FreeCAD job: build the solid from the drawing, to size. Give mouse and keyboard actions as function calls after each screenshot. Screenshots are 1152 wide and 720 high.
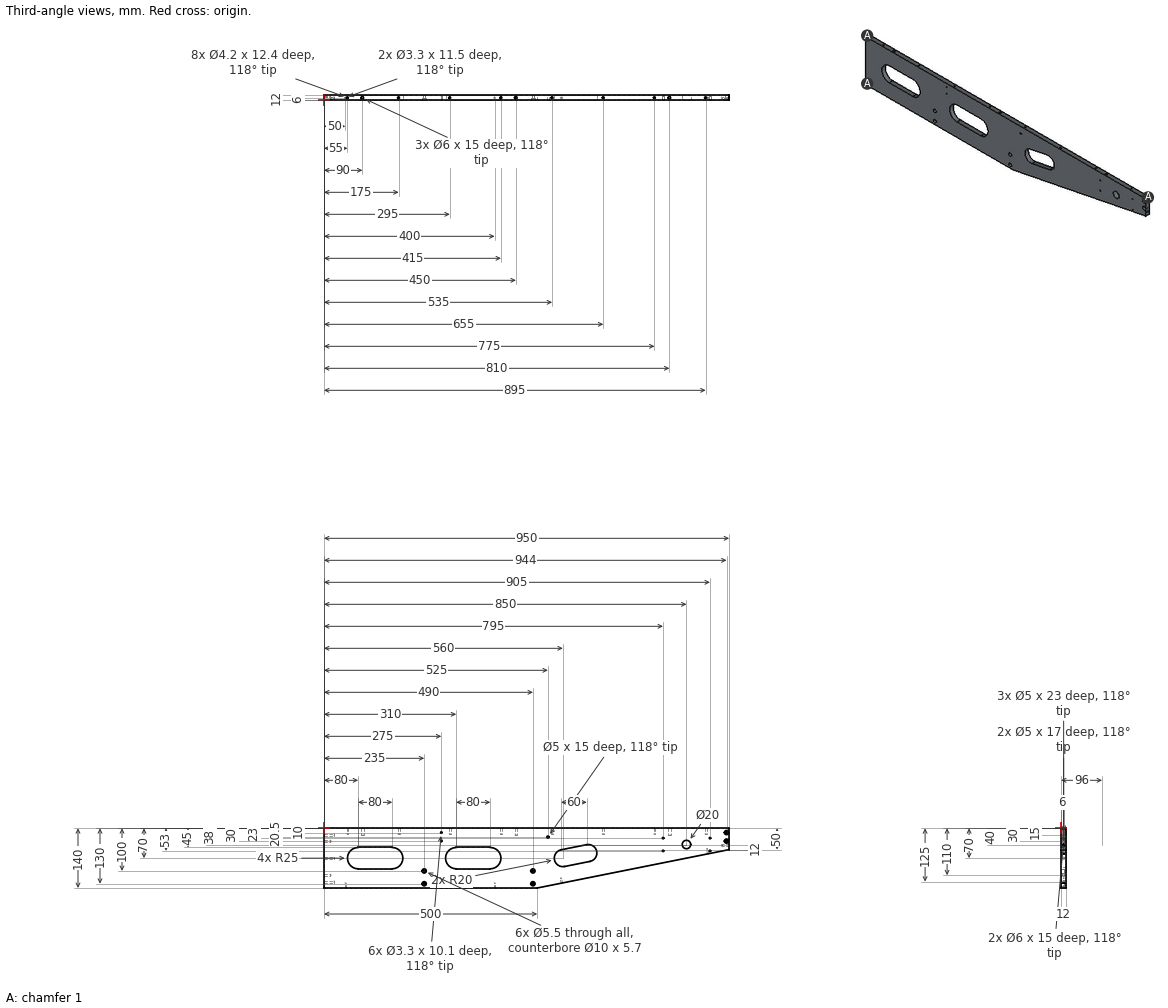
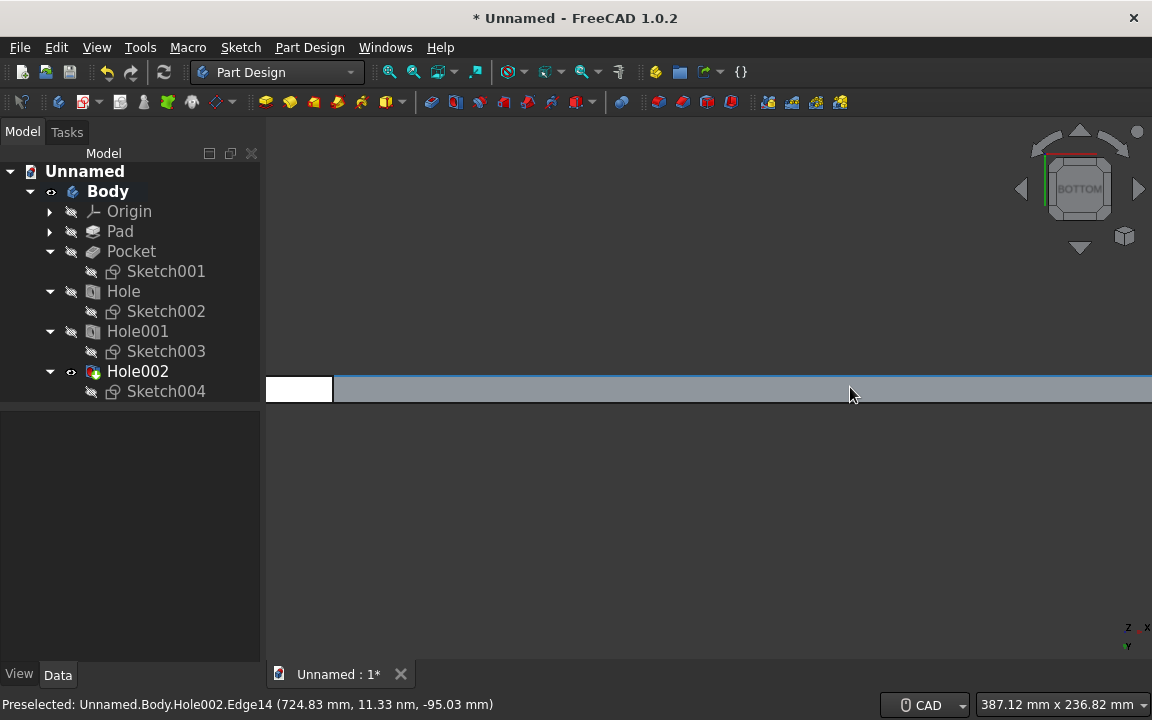
click(848, 389)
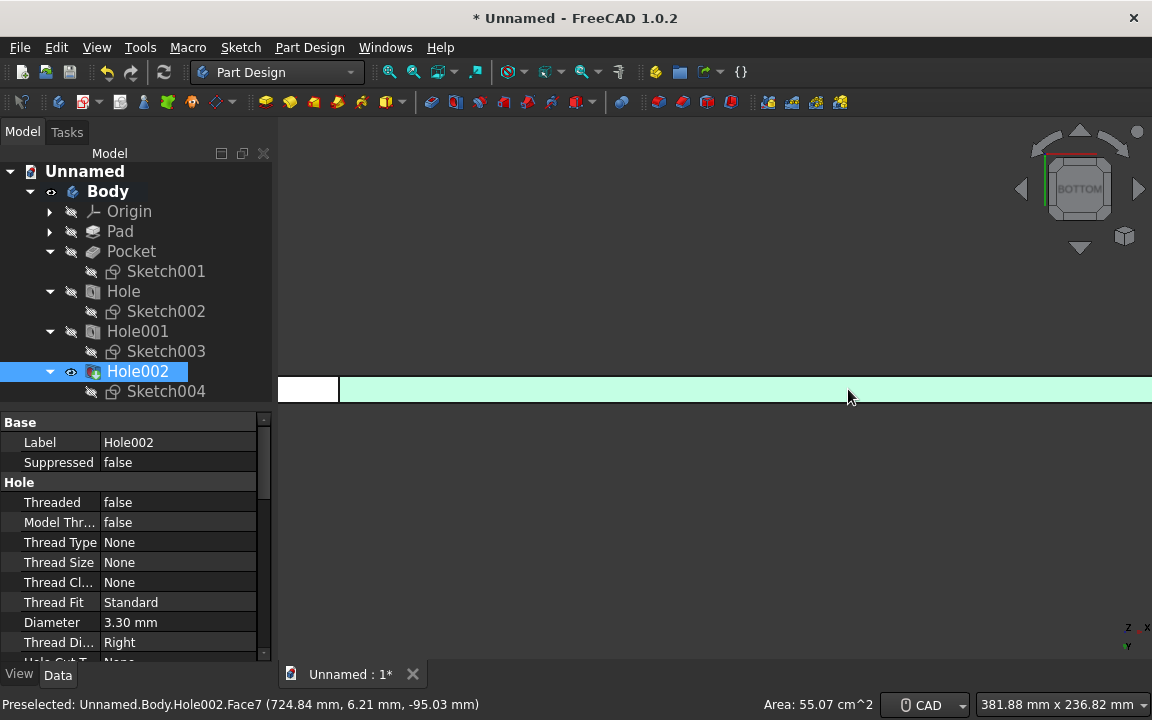
click(84, 102)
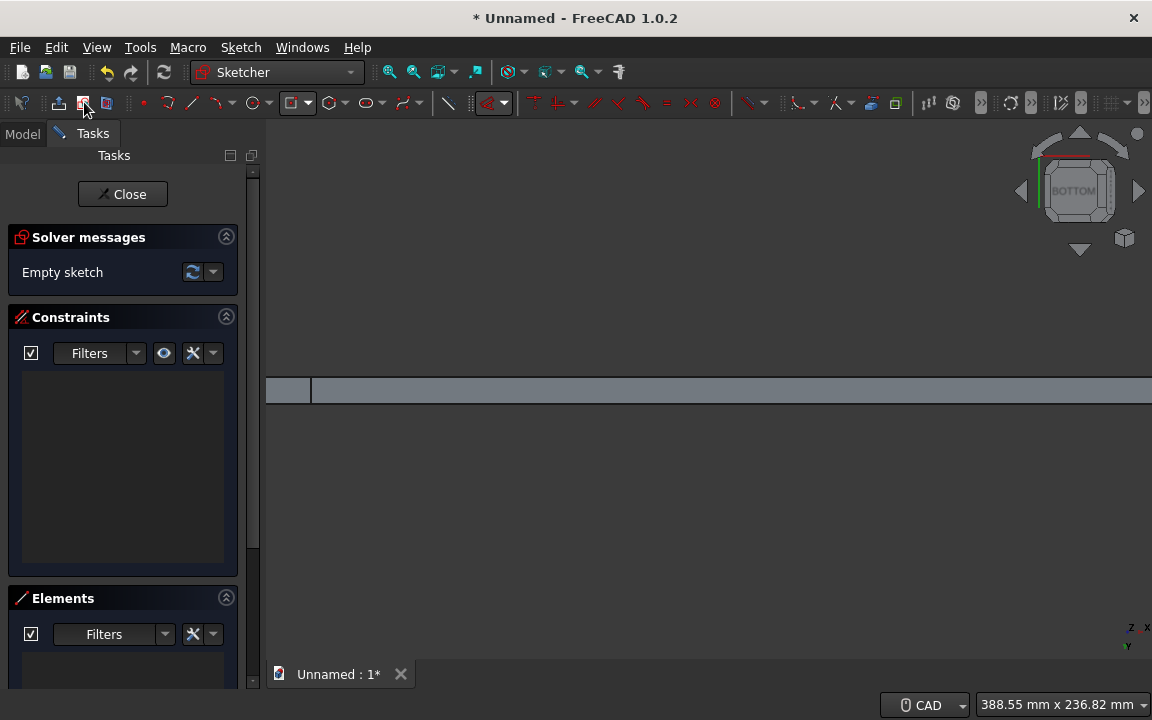
scroll(768, 390, down, 7)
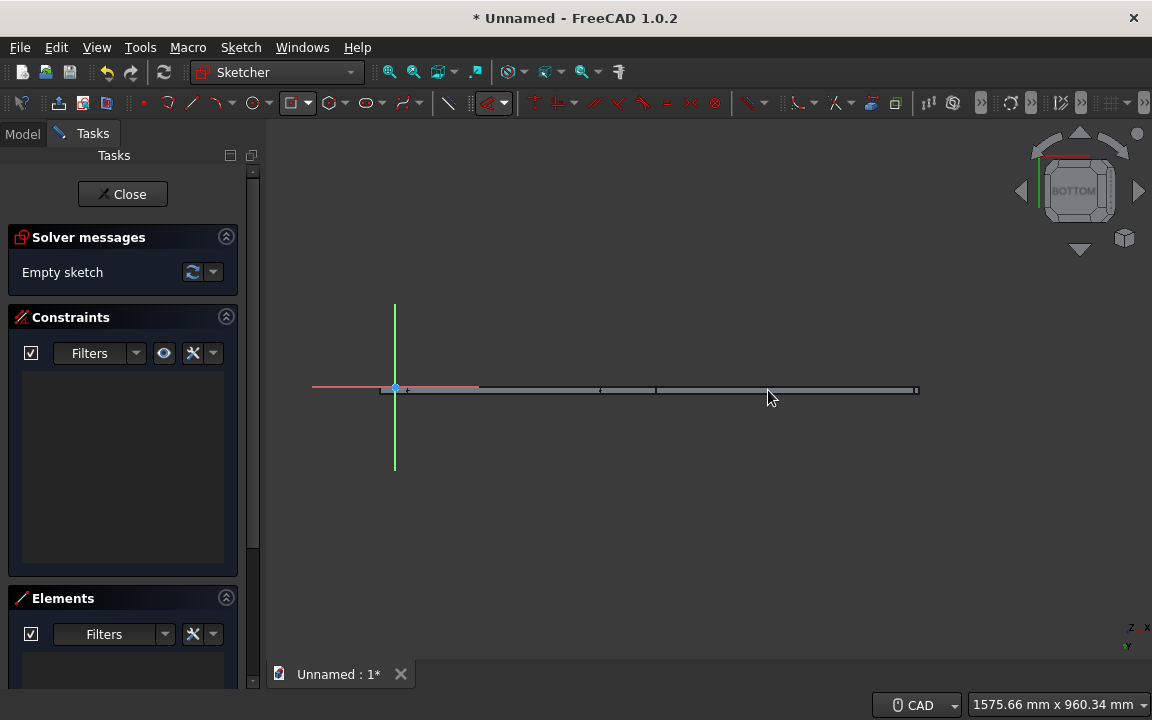
key(g)
key(c)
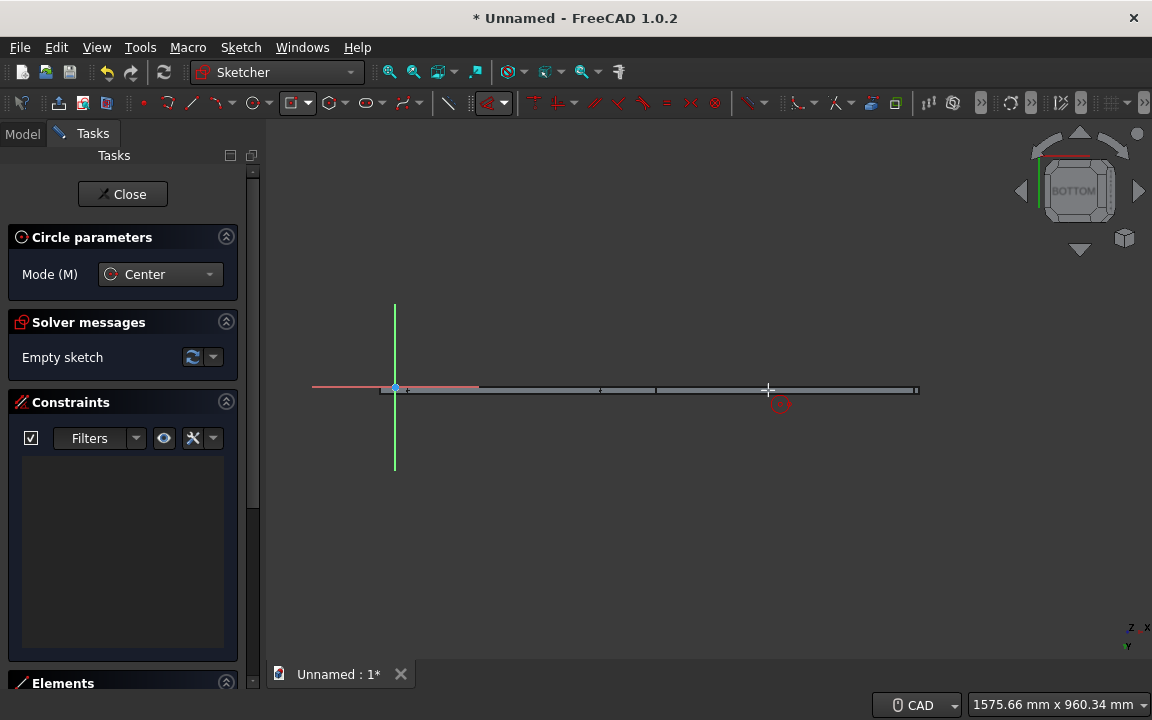
scroll(886, 391, up, 16)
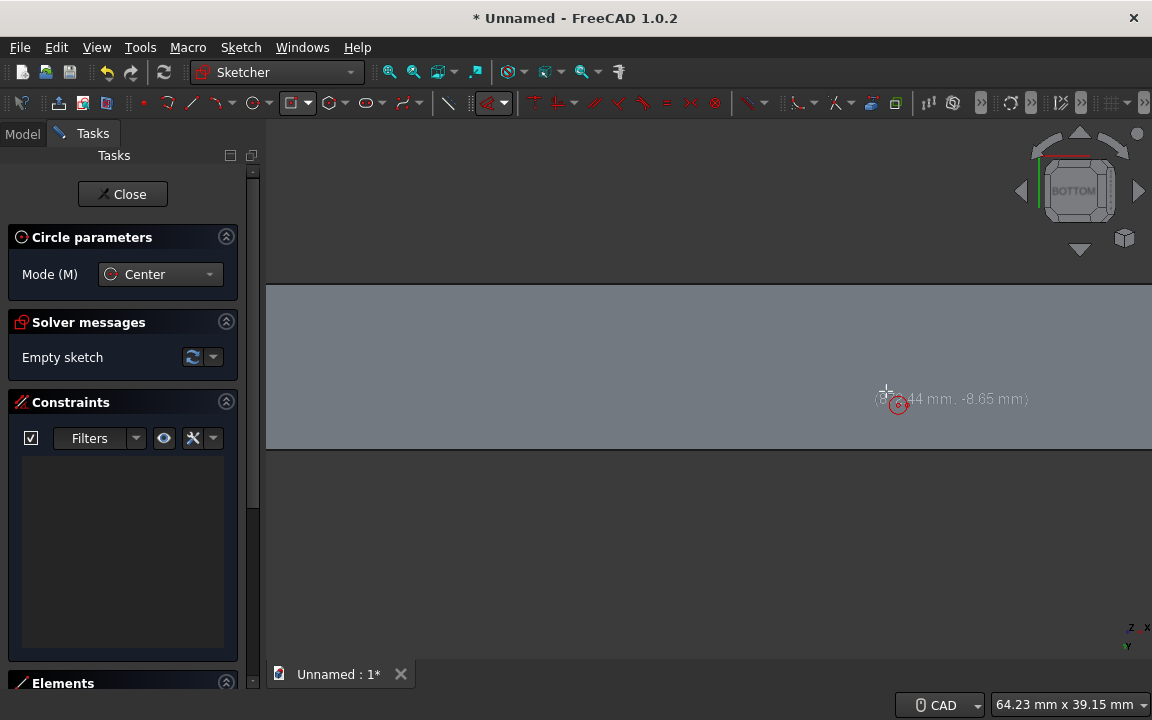
scroll(943, 392, down, 15)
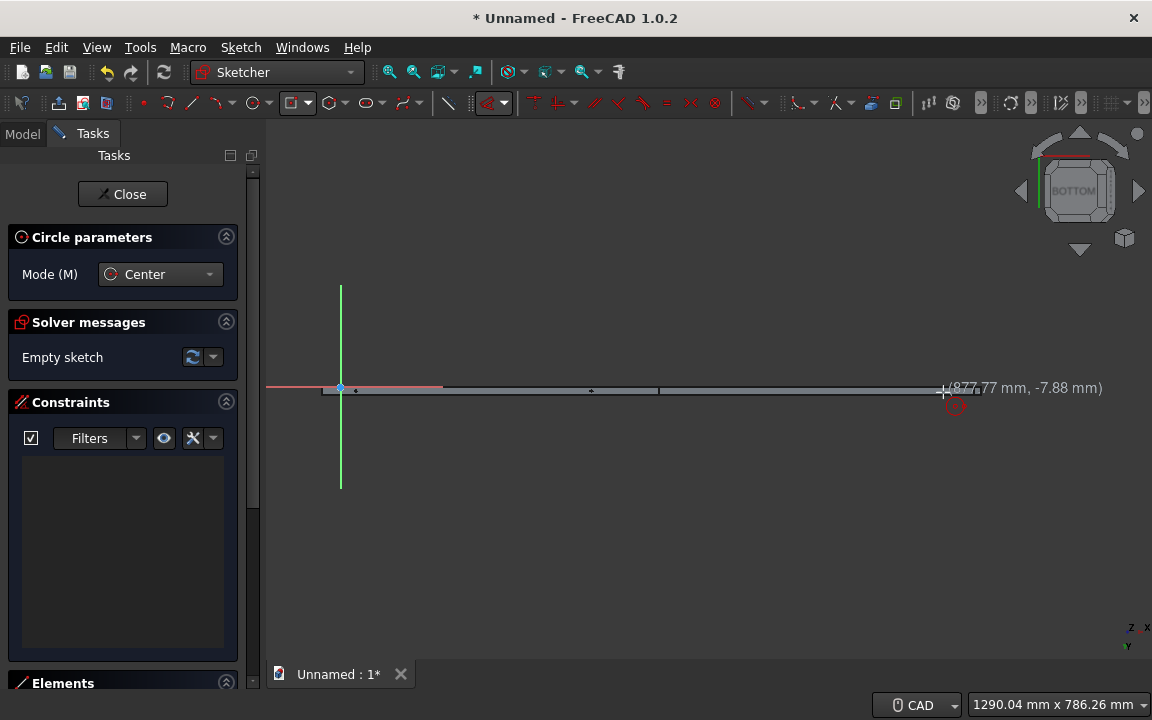
scroll(940, 391, up, 7)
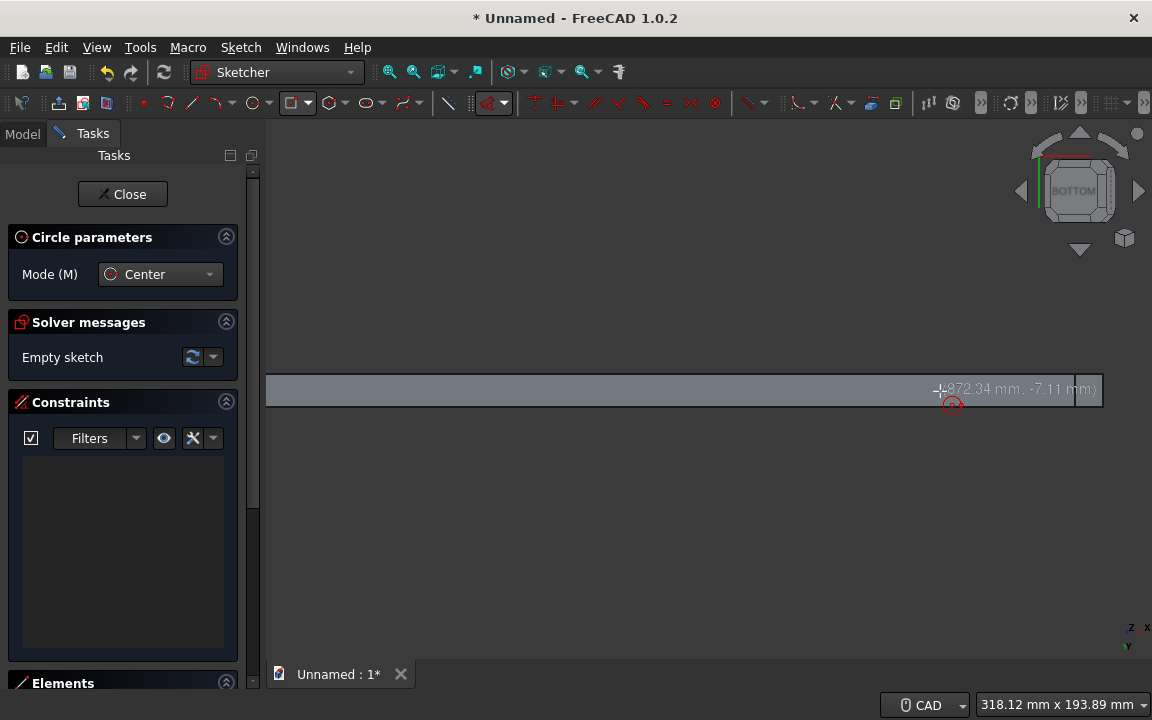
click(936, 390)
move(939, 394)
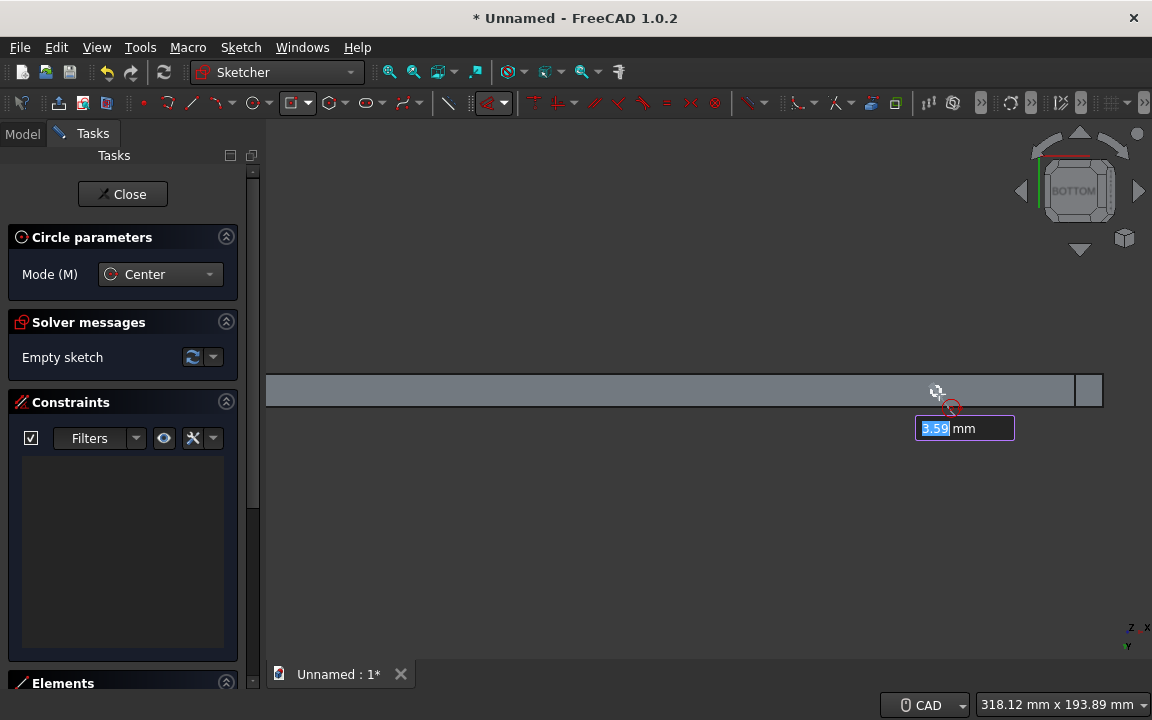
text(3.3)
key(Return)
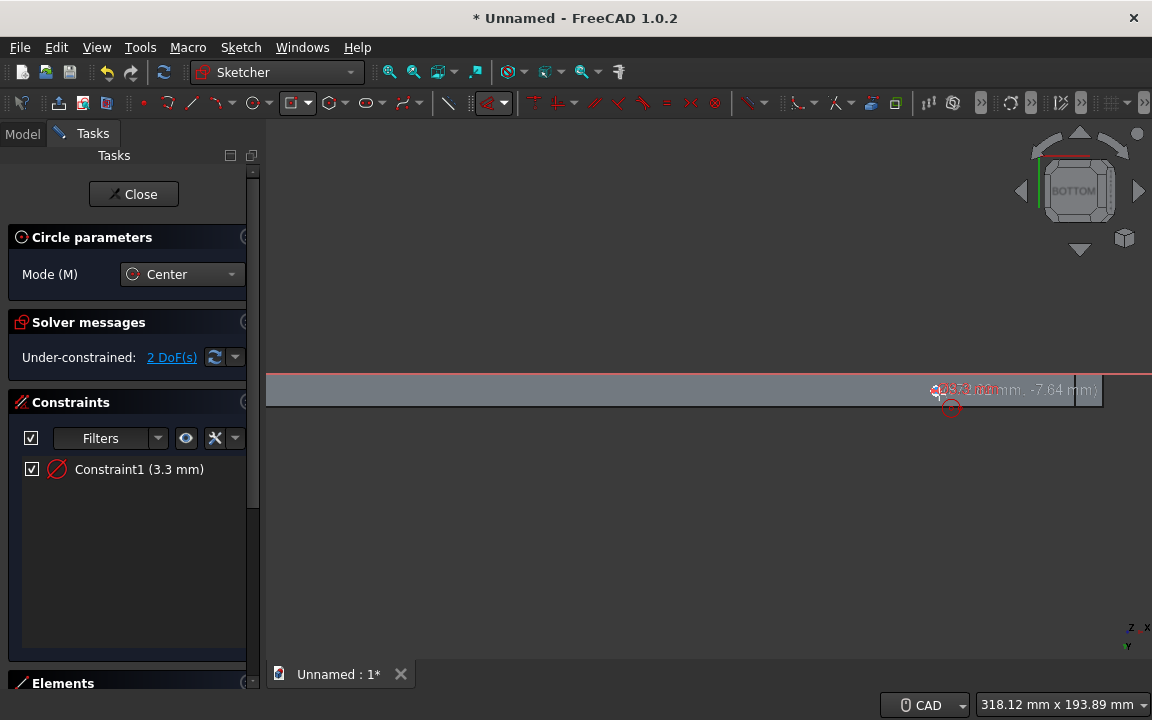
scroll(872, 390, down, 8)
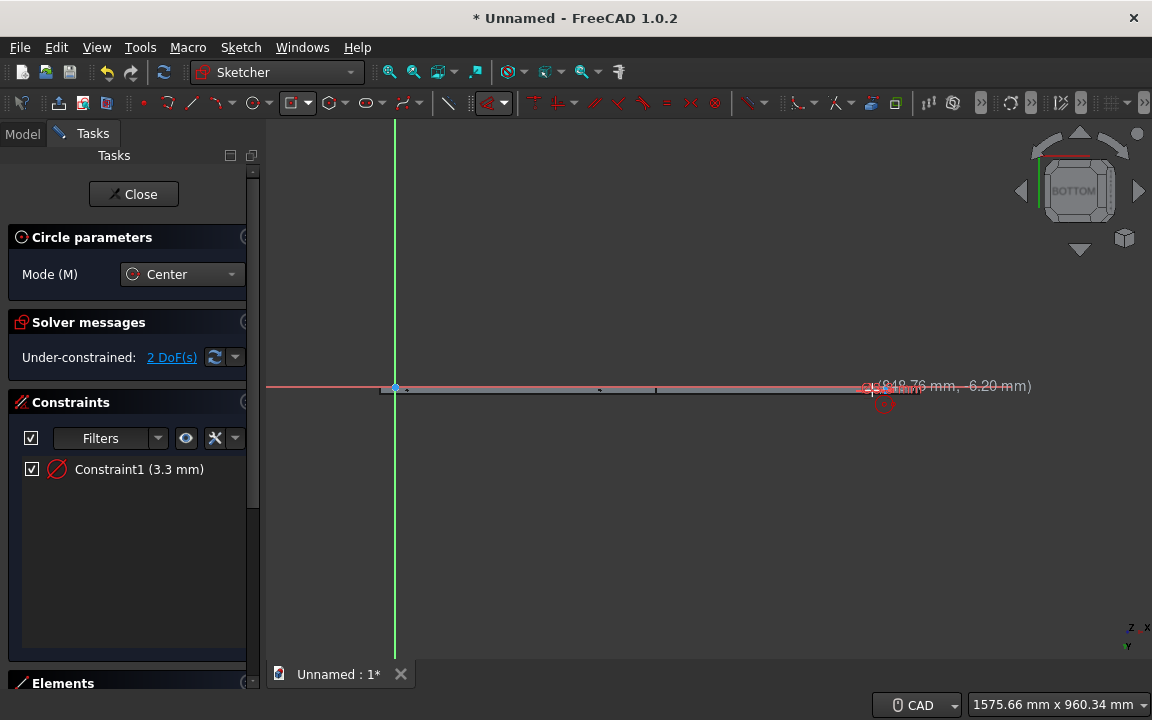
scroll(689, 390, up, 16)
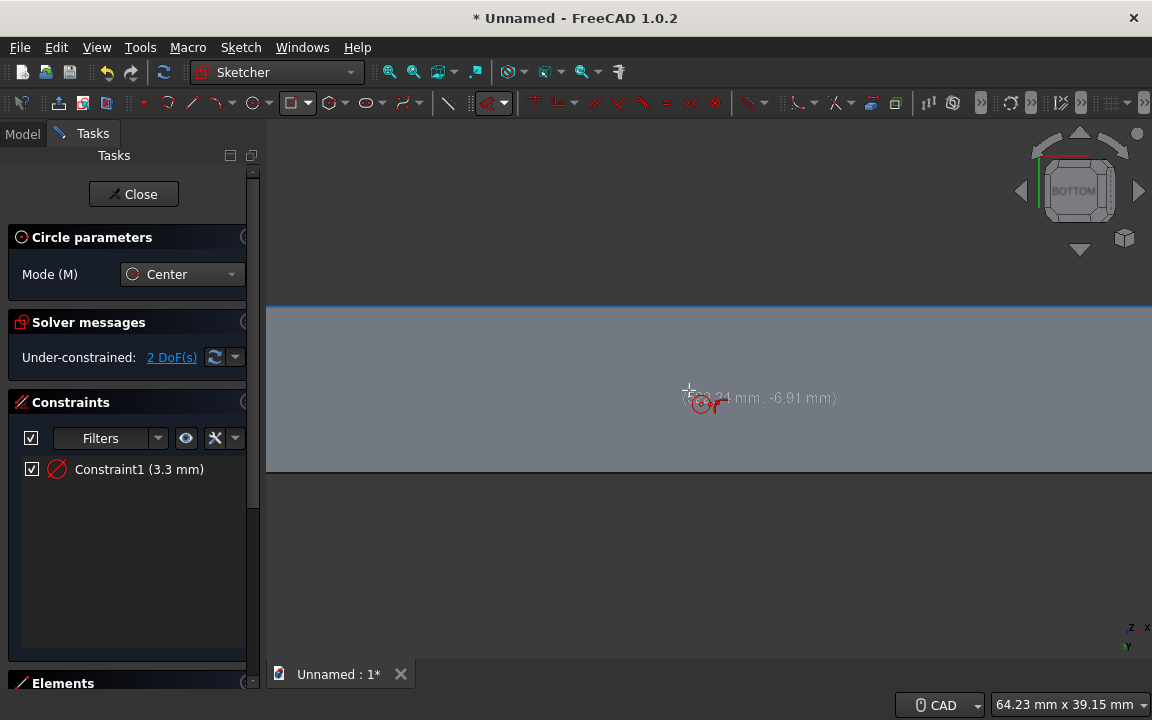
scroll(700, 391, down, 15)